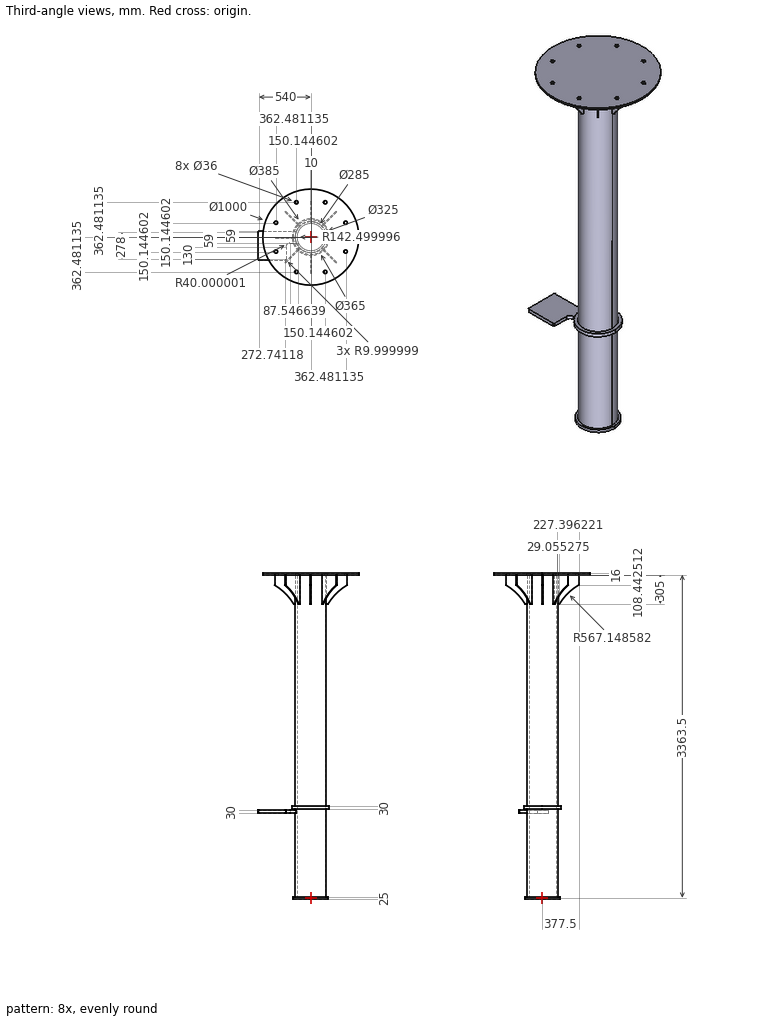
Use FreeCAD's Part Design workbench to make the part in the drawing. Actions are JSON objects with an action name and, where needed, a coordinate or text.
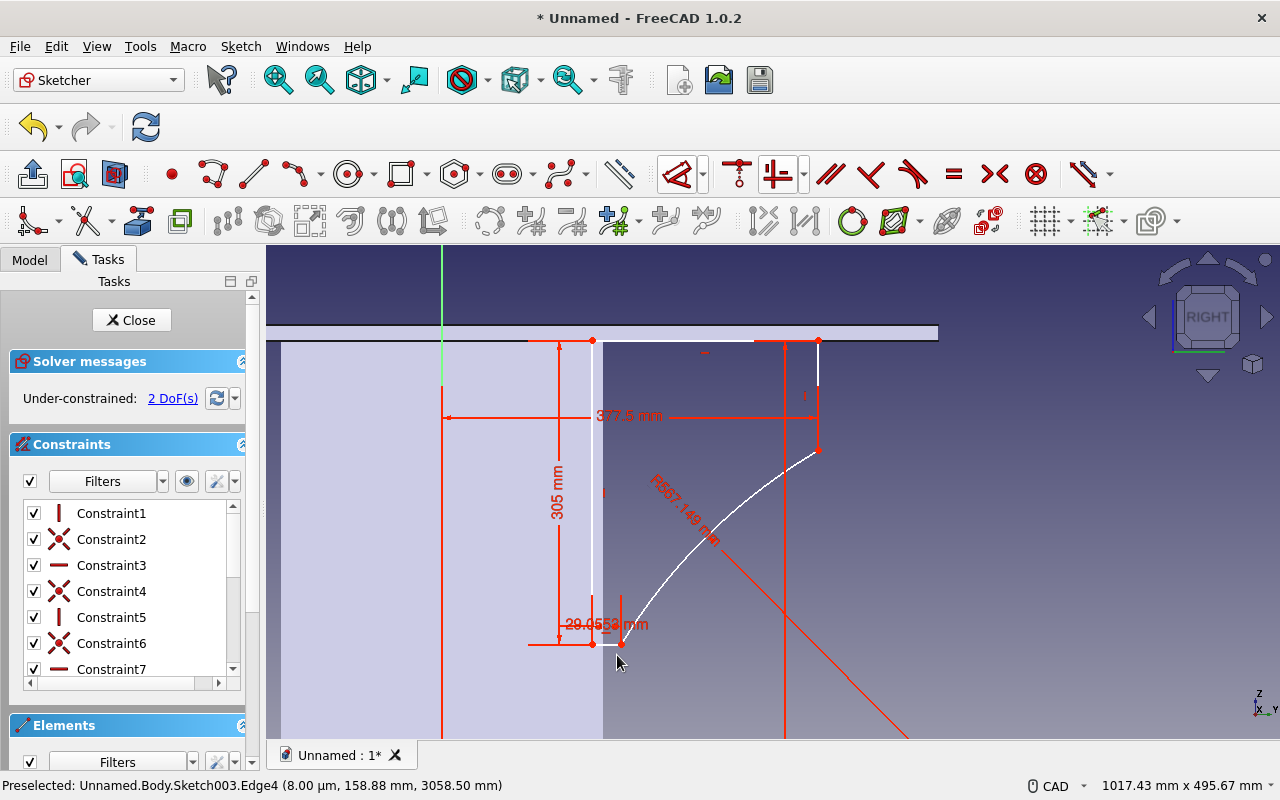
{"action": "left_click", "coordinate": [818, 418]}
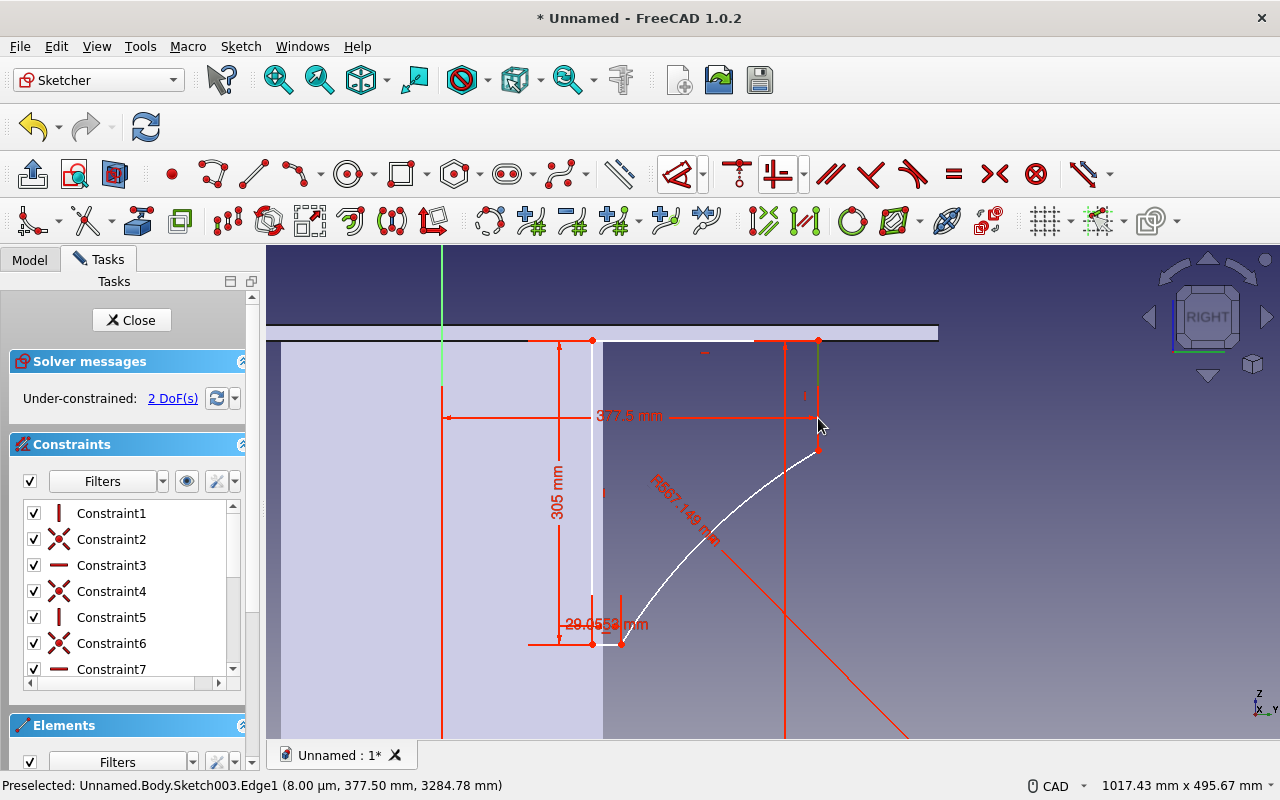
{"action": "key", "text": "i"}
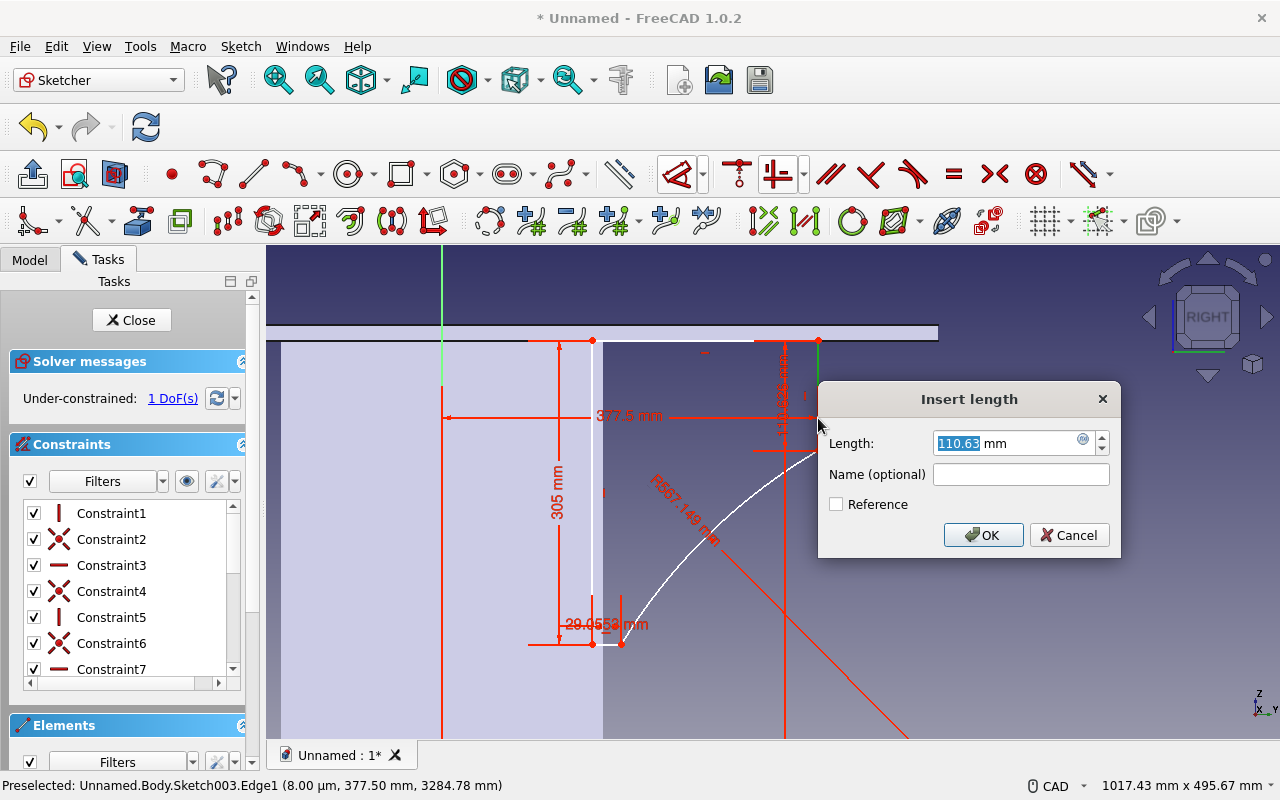
{"action": "type", "text": "108.442512"}
{"action": "key", "text": "Return"}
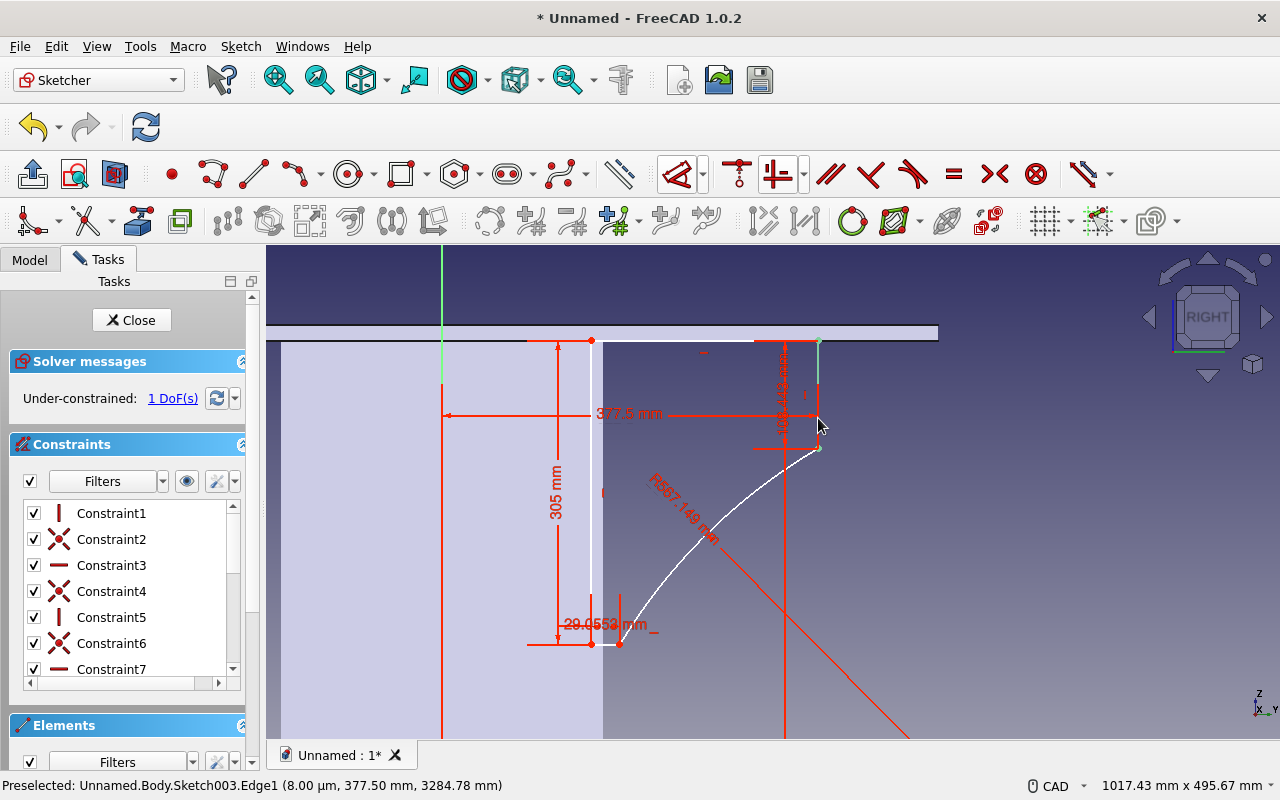
{"action": "left_click", "coordinate": [750, 341]}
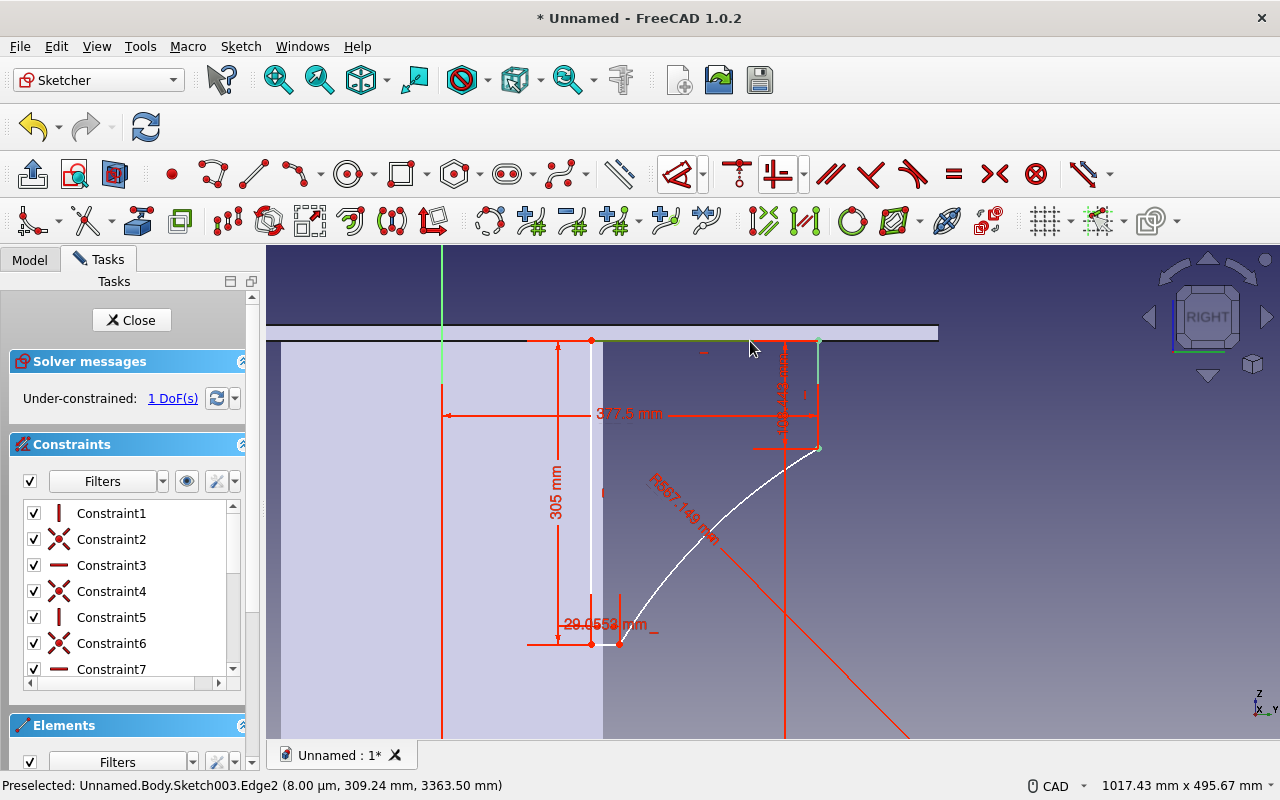
{"action": "left_click", "coordinate": [702, 174]}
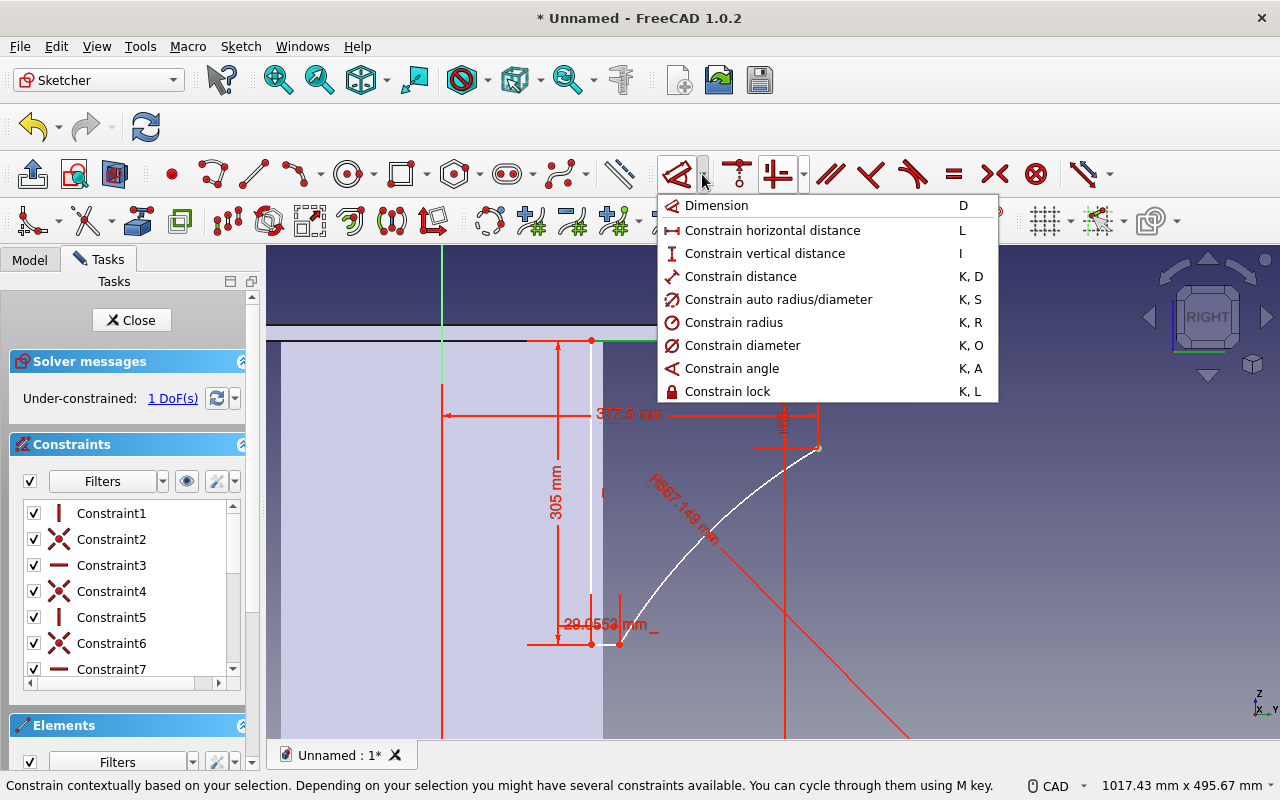
{"action": "left_click", "coordinate": [828, 230]}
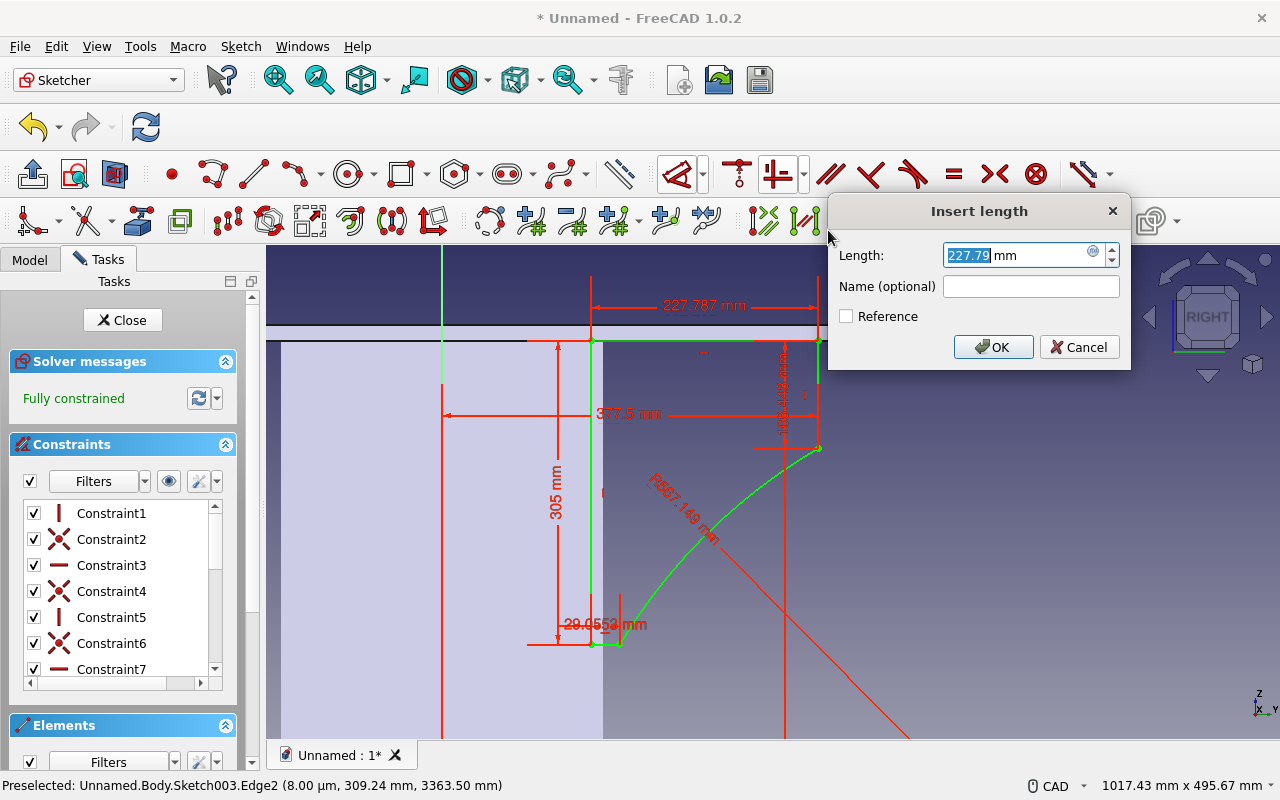
{"action": "type", "text": "227.396221"}
{"action": "key", "text": "Return"}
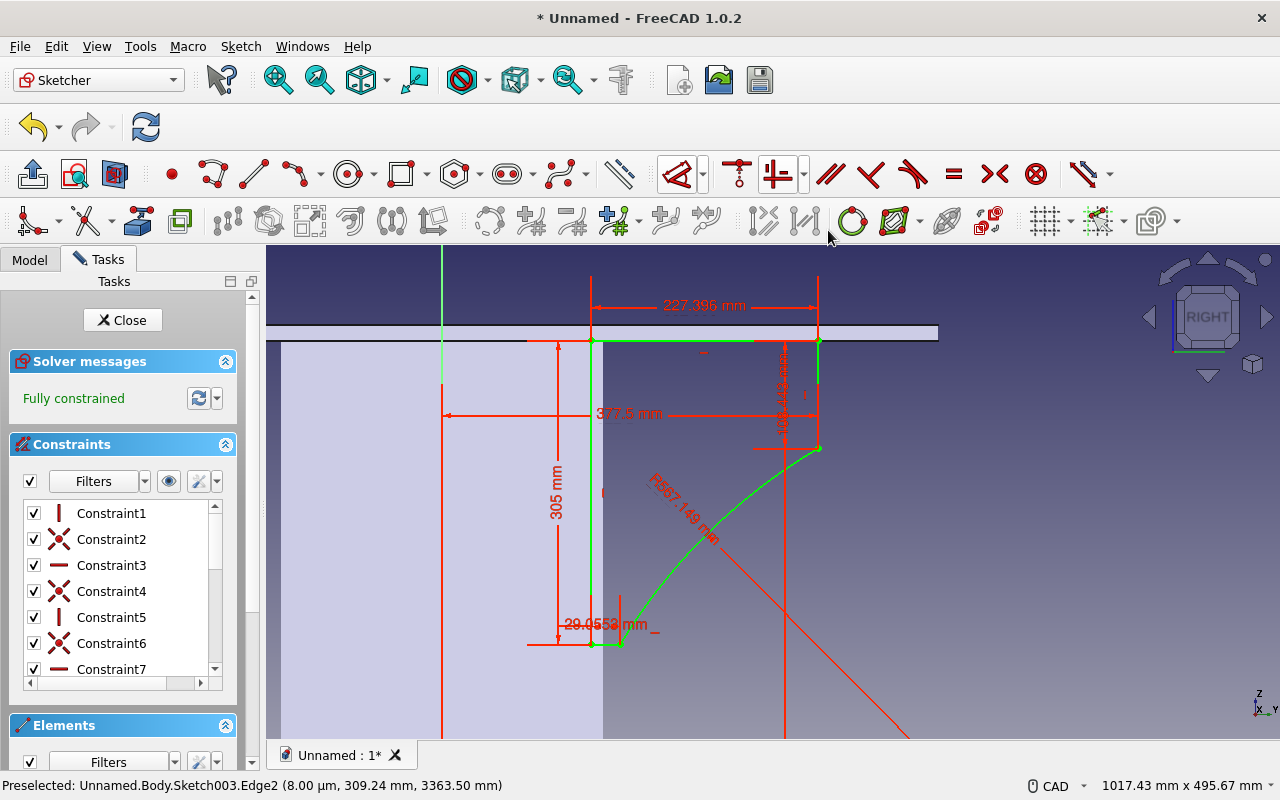
{"action": "left_click", "coordinate": [123, 320]}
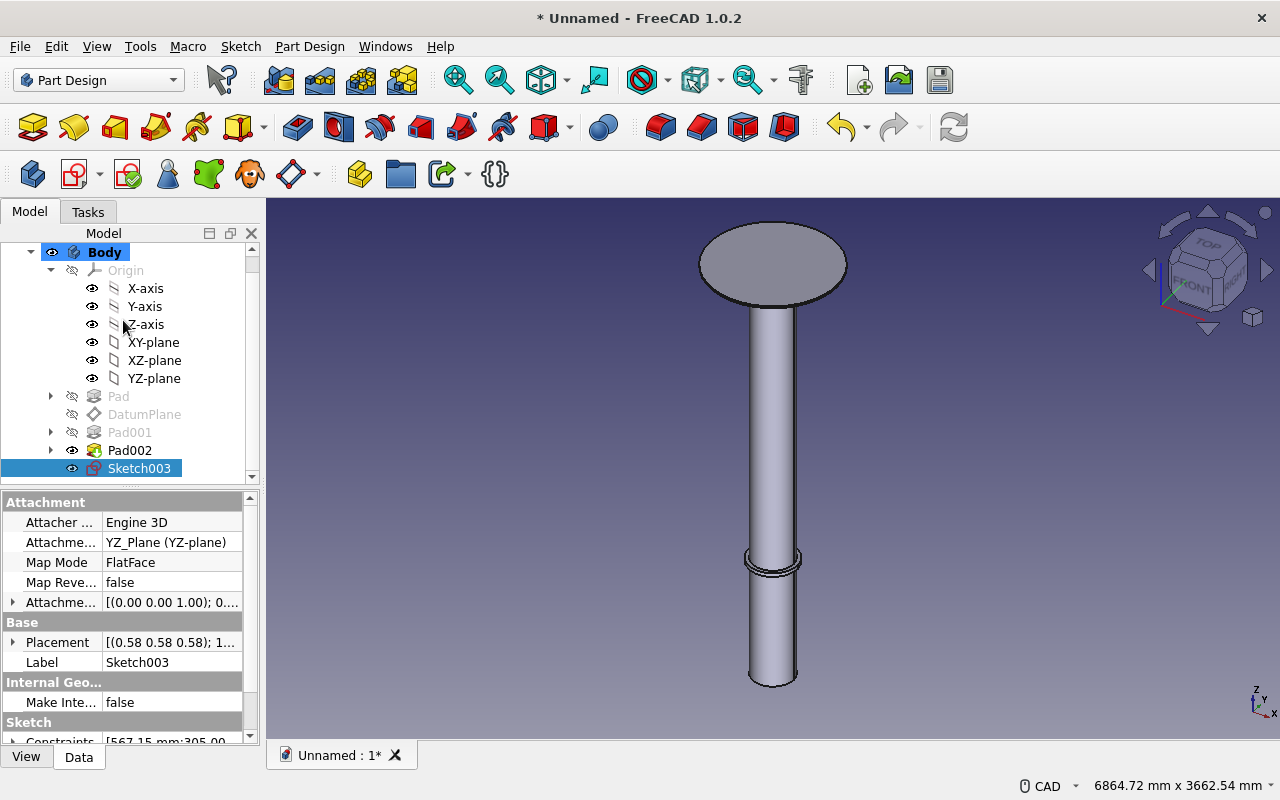
{"action": "left_click", "coordinate": [33, 128]}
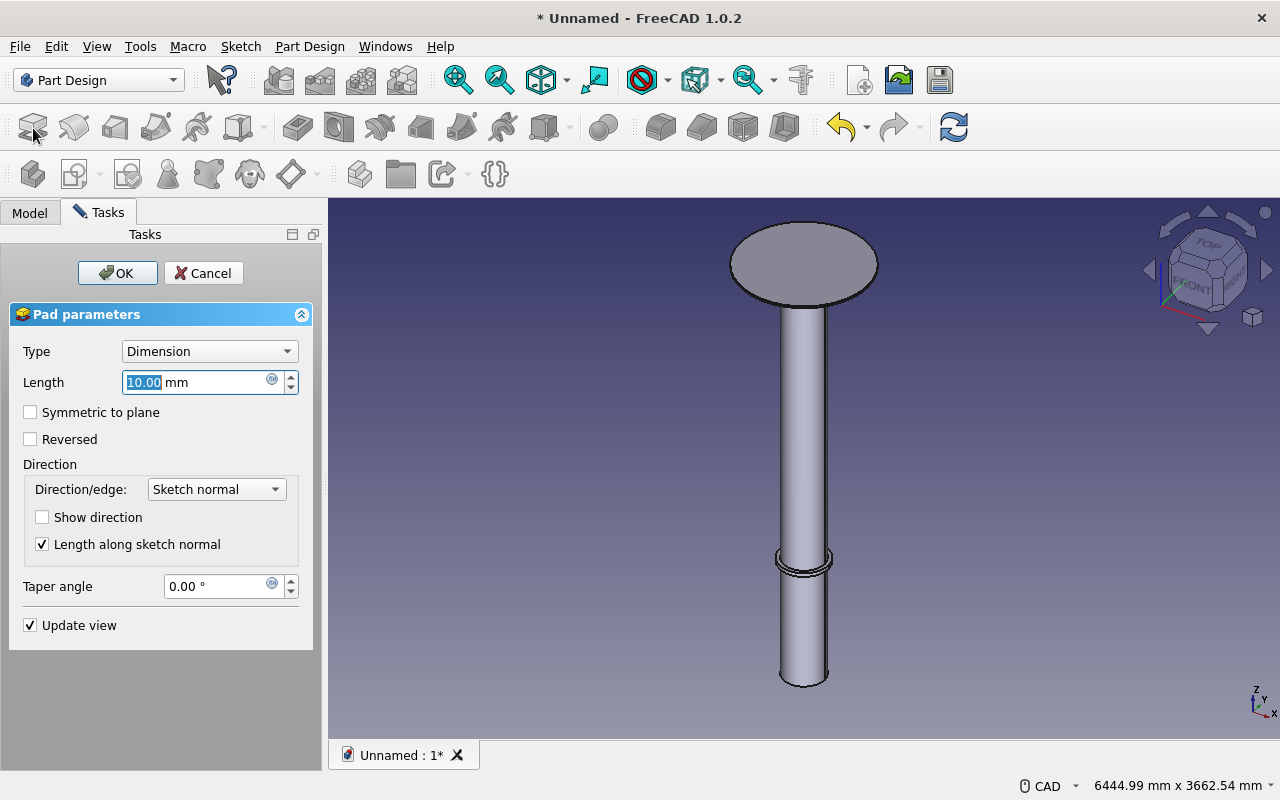
{"action": "type", "text": "10"}
{"action": "key", "text": "Tab"}